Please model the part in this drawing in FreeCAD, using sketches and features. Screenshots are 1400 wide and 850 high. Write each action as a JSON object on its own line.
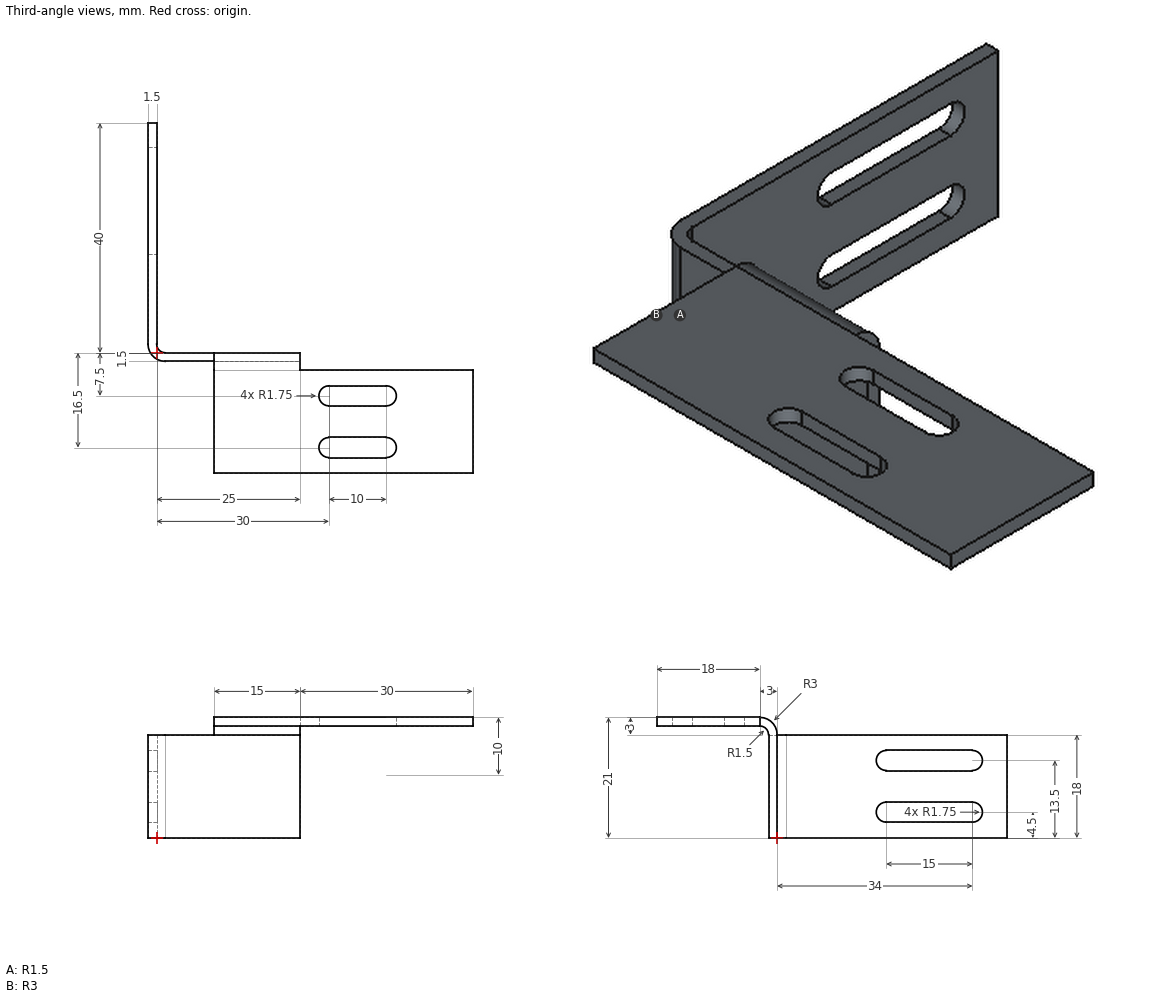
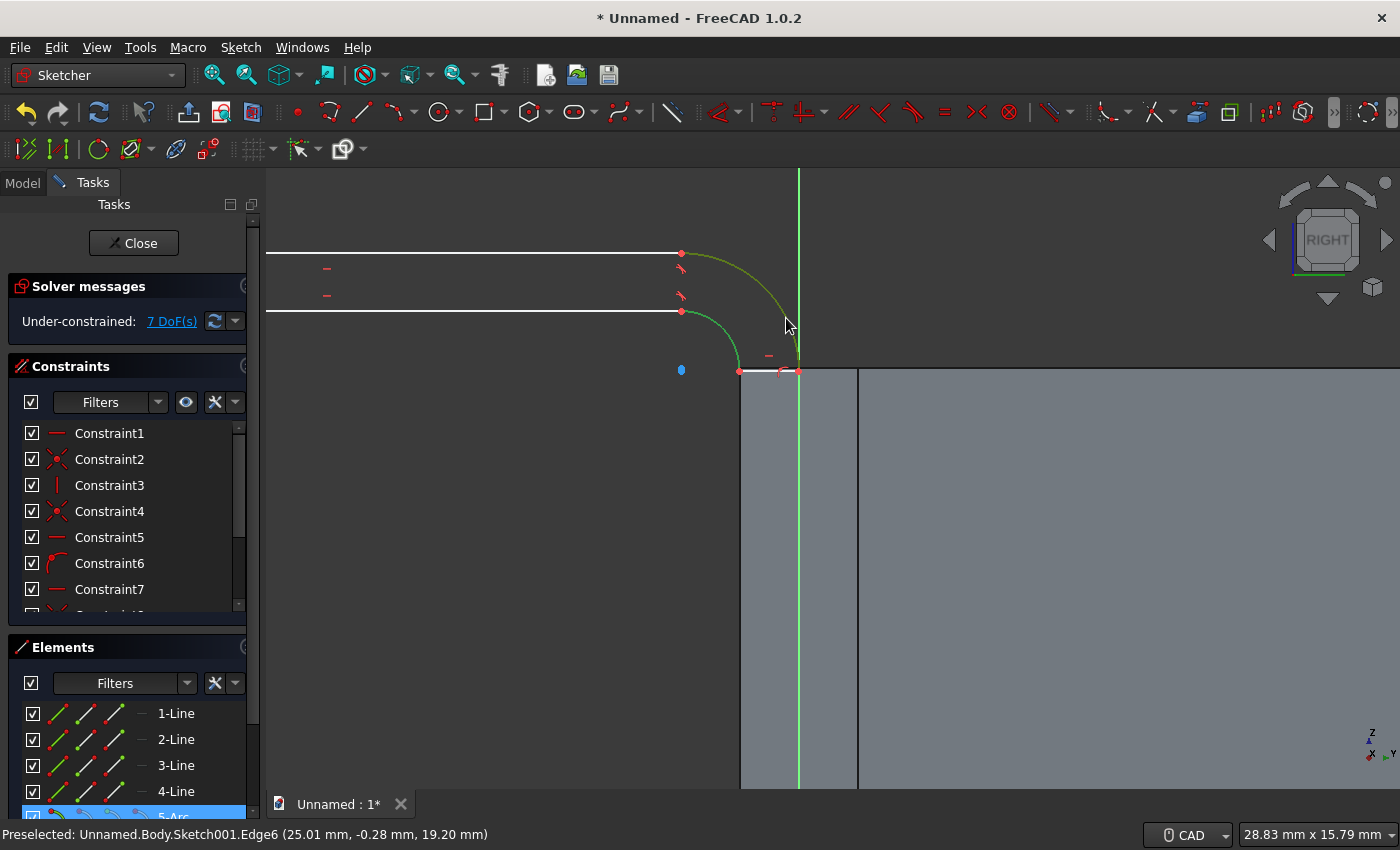
{"action": "key", "text": "c"}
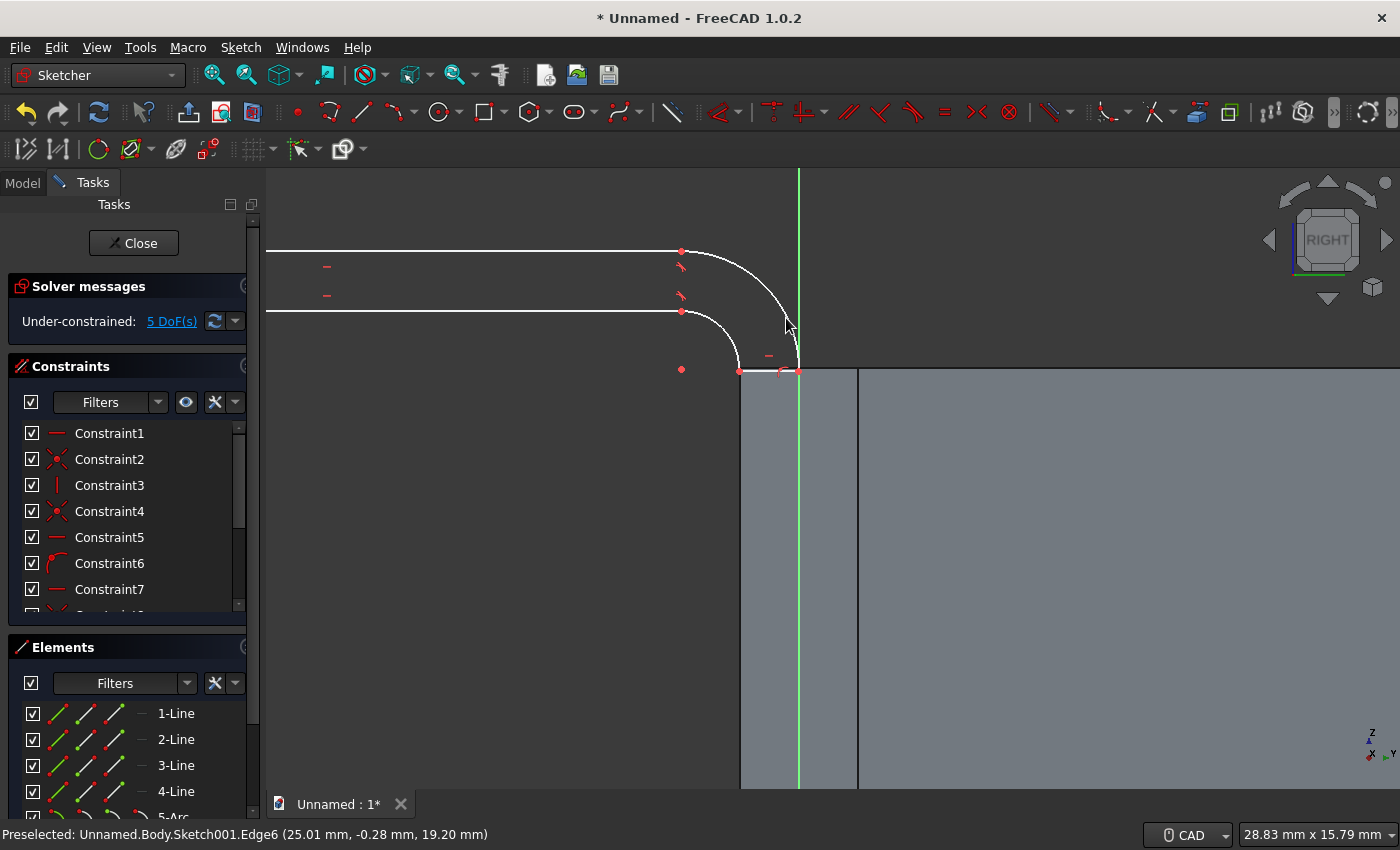
{"action": "key", "text": "d"}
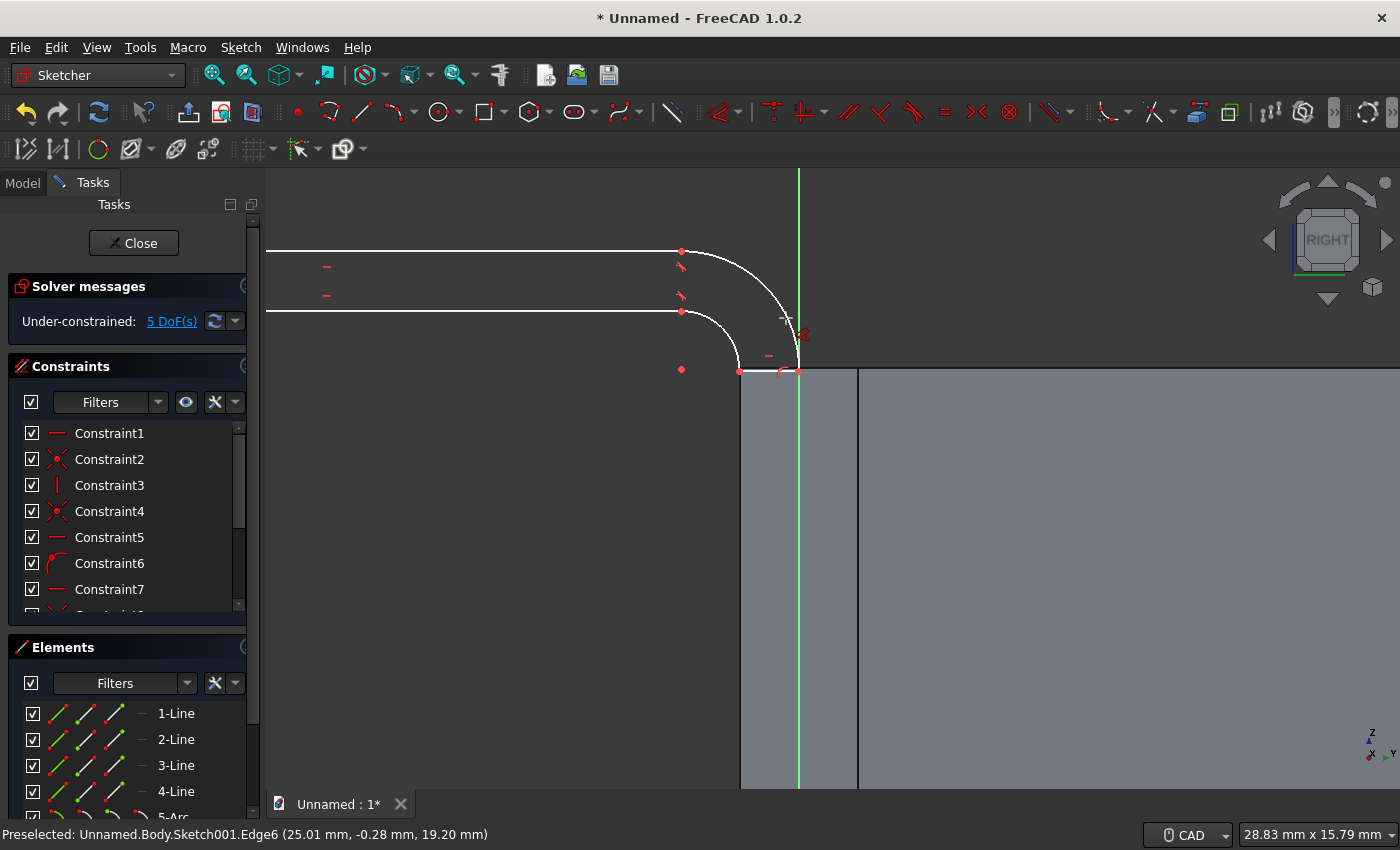
{"action": "left_click", "coordinate": [733, 344]}
{"action": "left_click", "coordinate": [762, 330]}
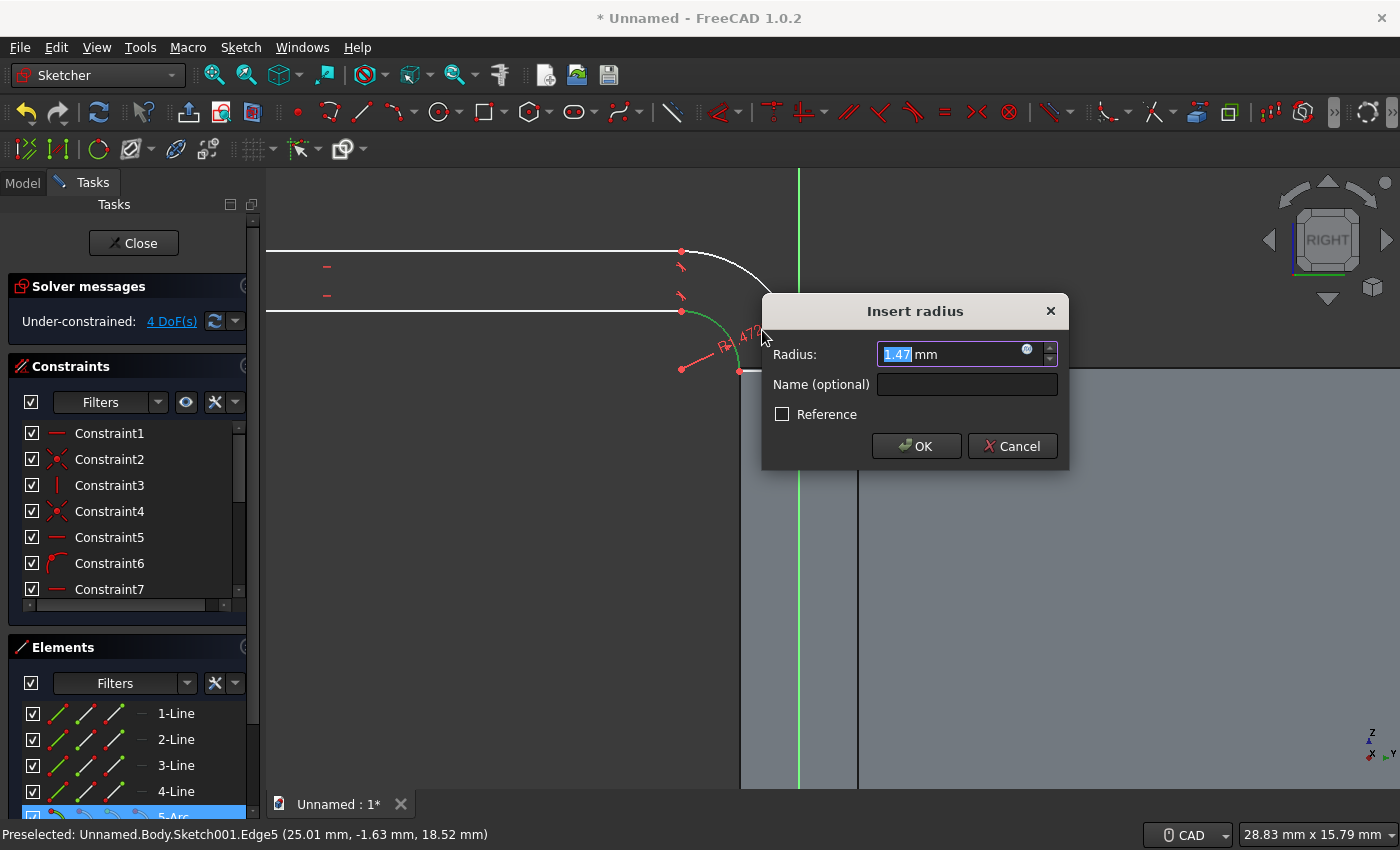
{"action": "type", "text": "1.5"}
{"action": "key", "text": "Return"}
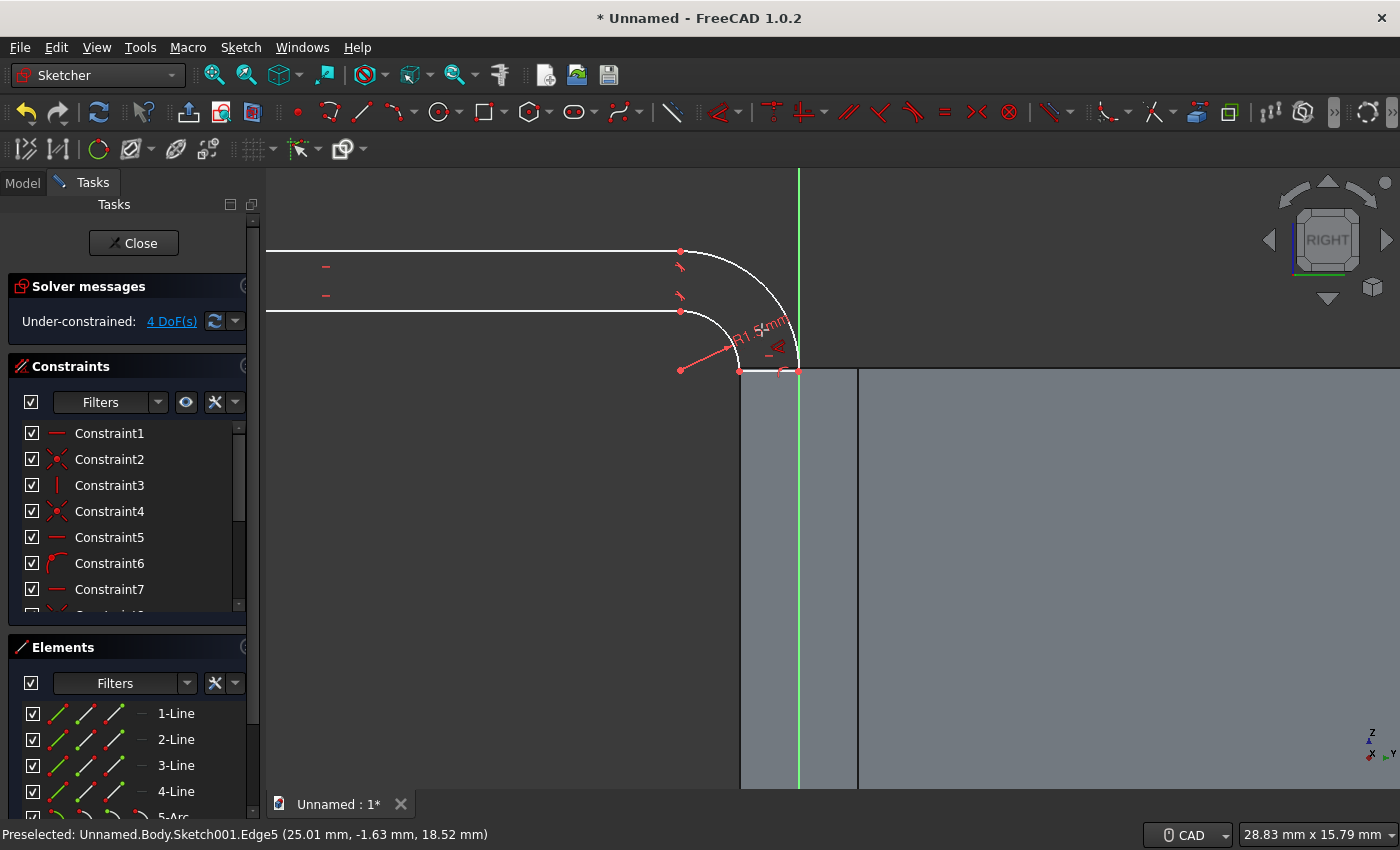
{"action": "left_click", "coordinate": [786, 317]}
{"action": "left_click", "coordinate": [815, 303]}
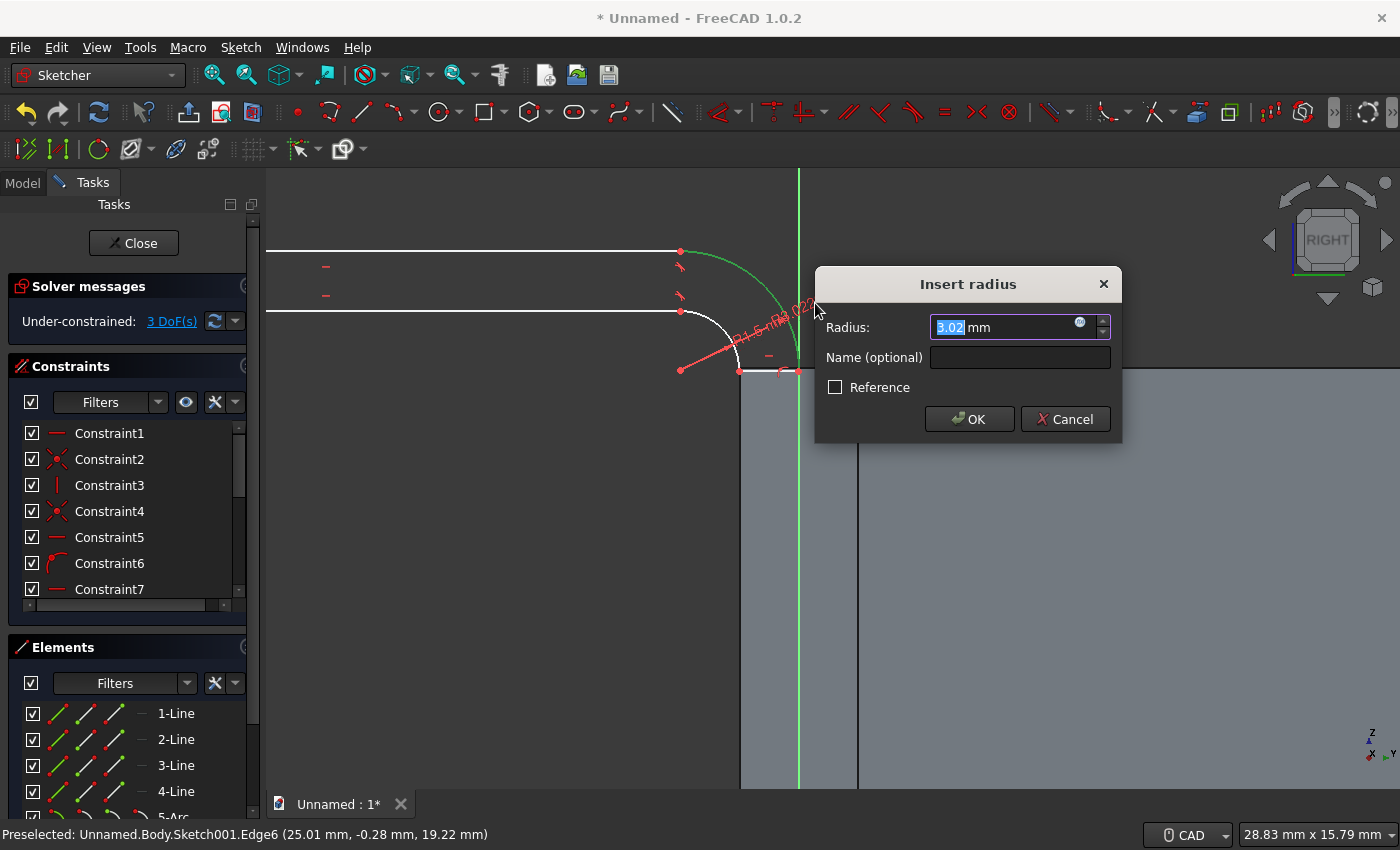
{"action": "type", "text": "3"}
{"action": "key", "text": "Return"}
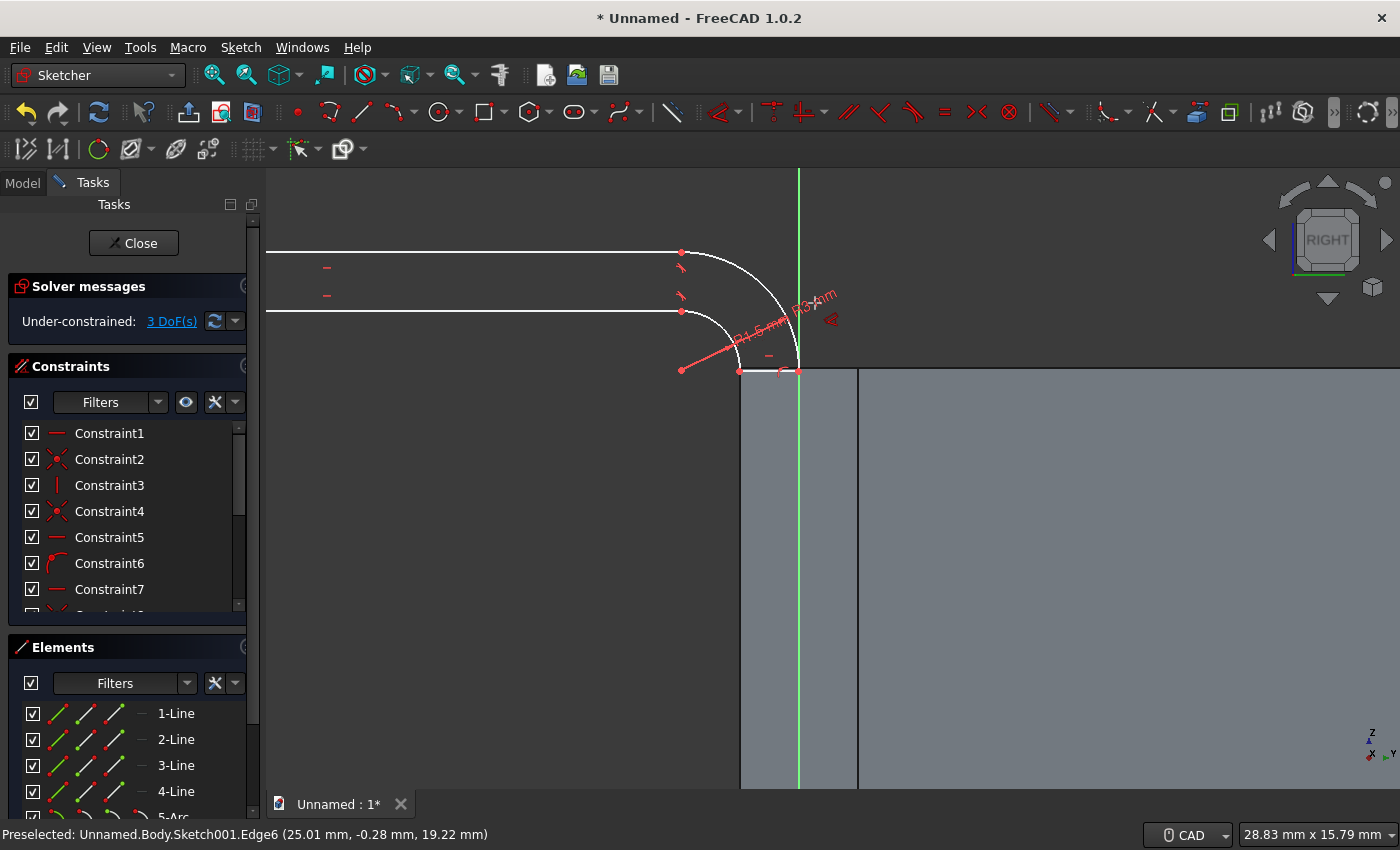
{"action": "left_click", "coordinate": [469, 252]}
{"action": "left_click", "coordinate": [488, 218]}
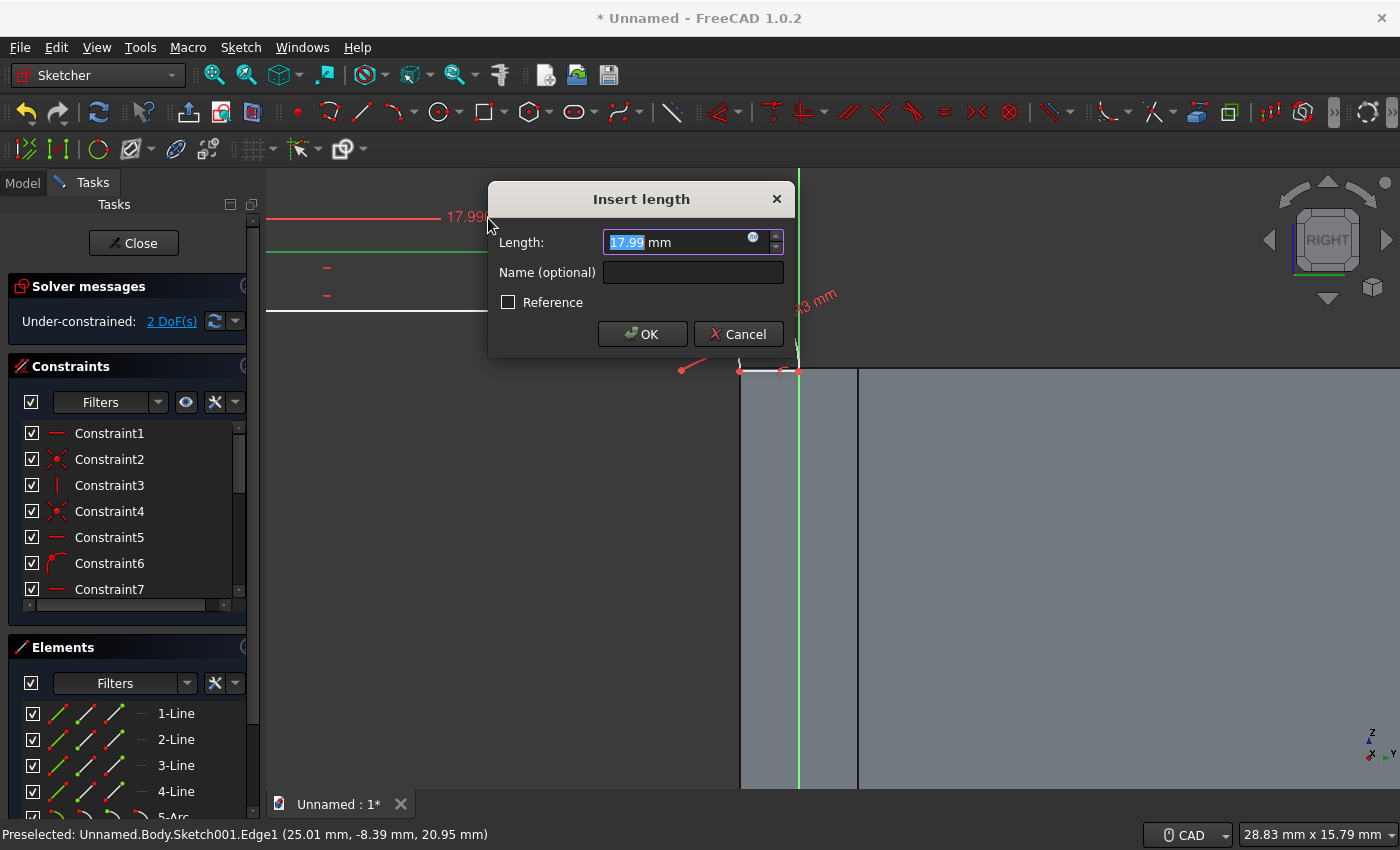
{"action": "type", "text": "18"}
{"action": "key", "text": "Return"}